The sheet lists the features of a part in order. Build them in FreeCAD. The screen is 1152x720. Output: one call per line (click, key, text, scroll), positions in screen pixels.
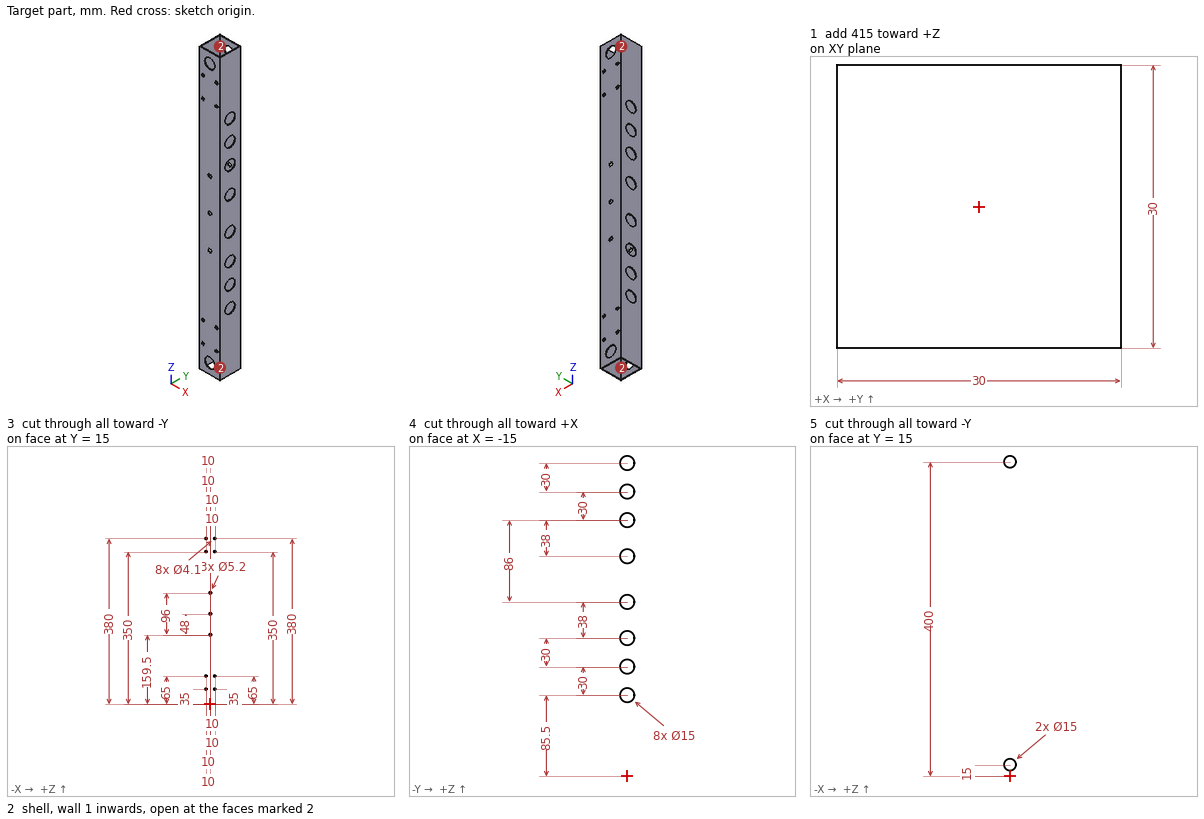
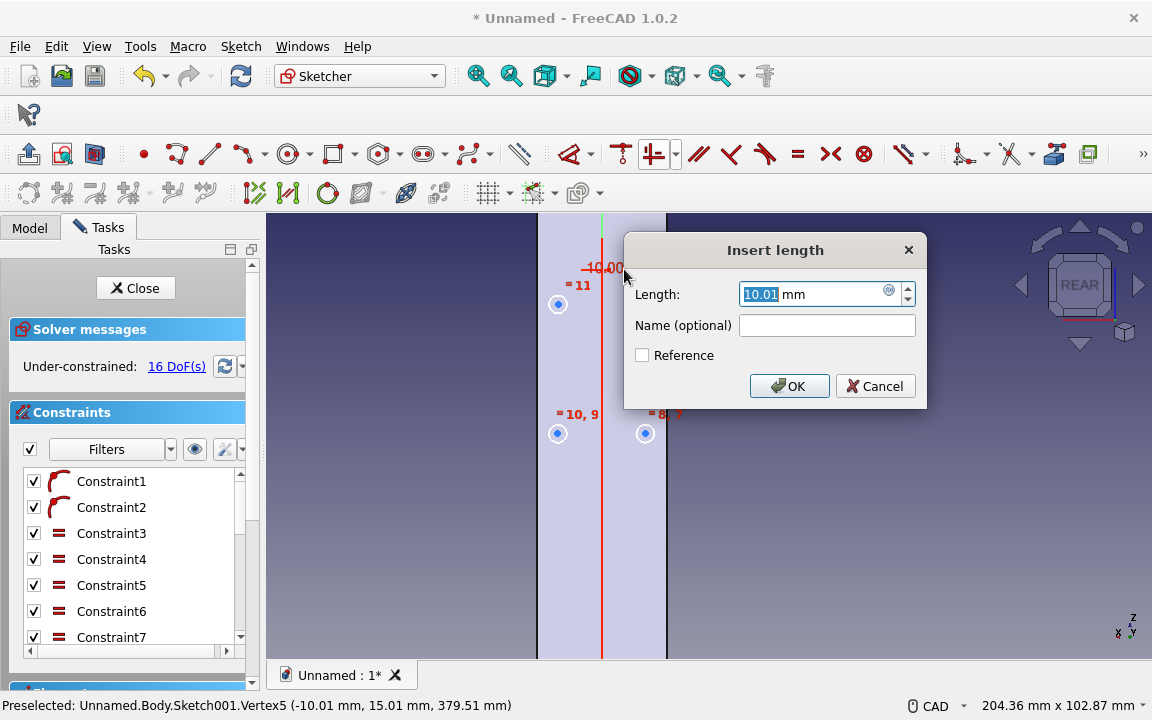
text(10)
key(Return)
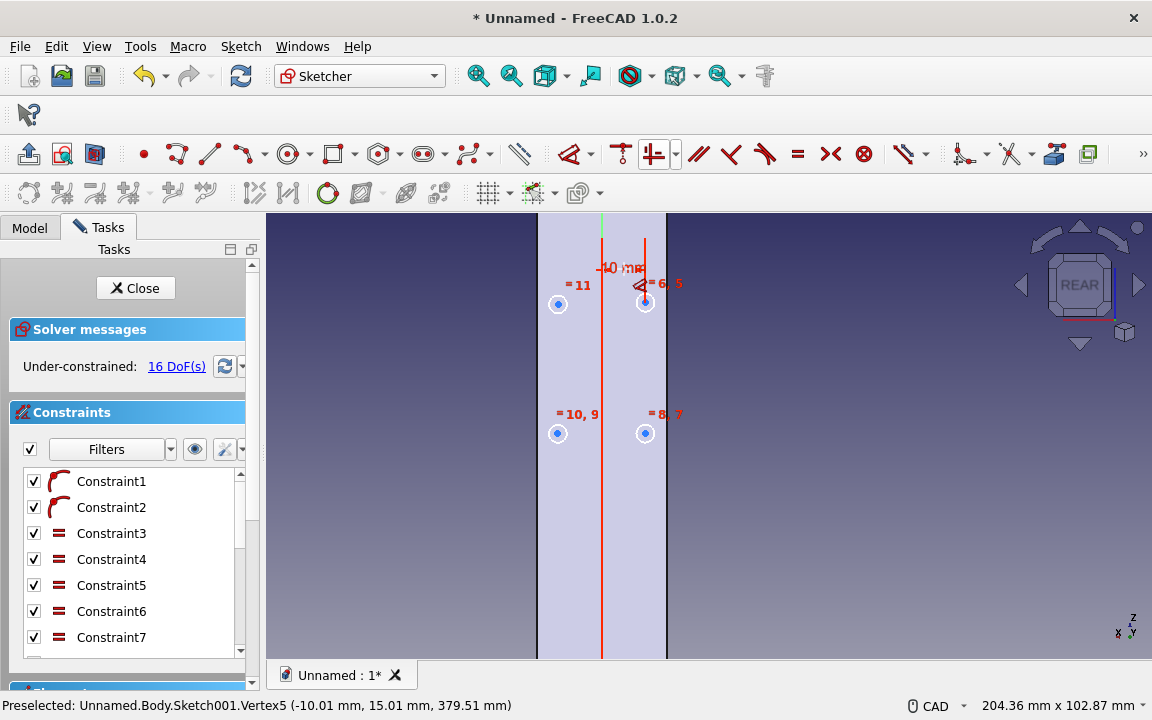
scroll(648, 301, down, 9)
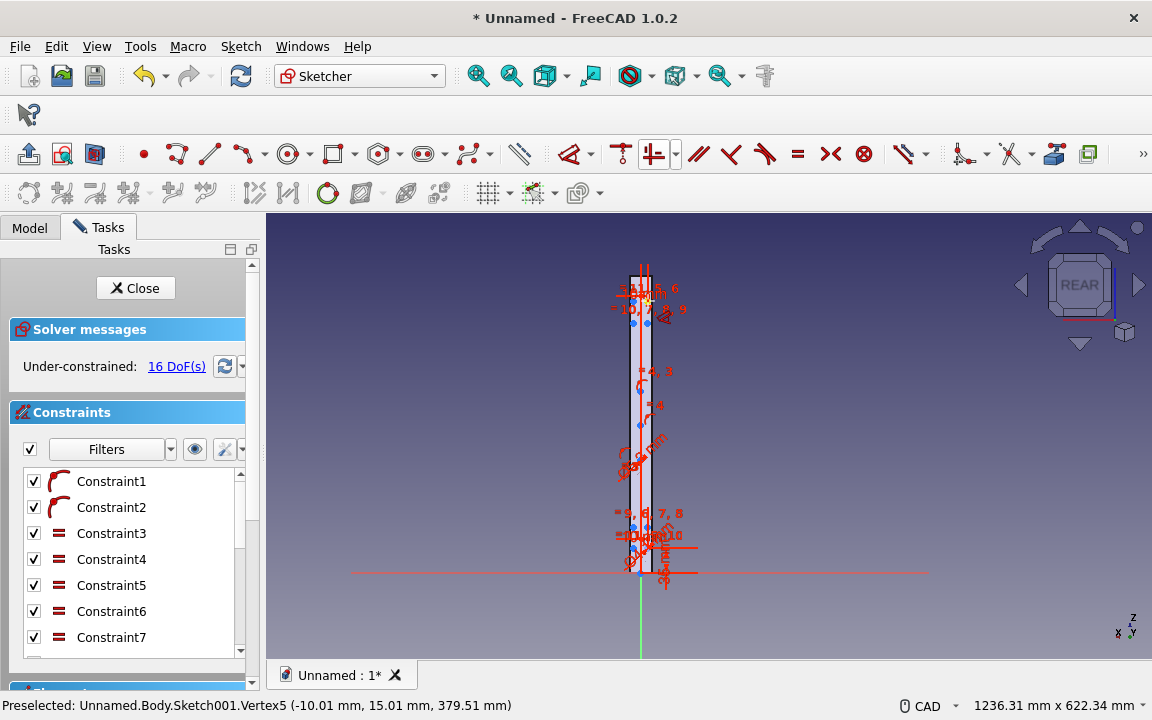
scroll(648, 527, up, 9)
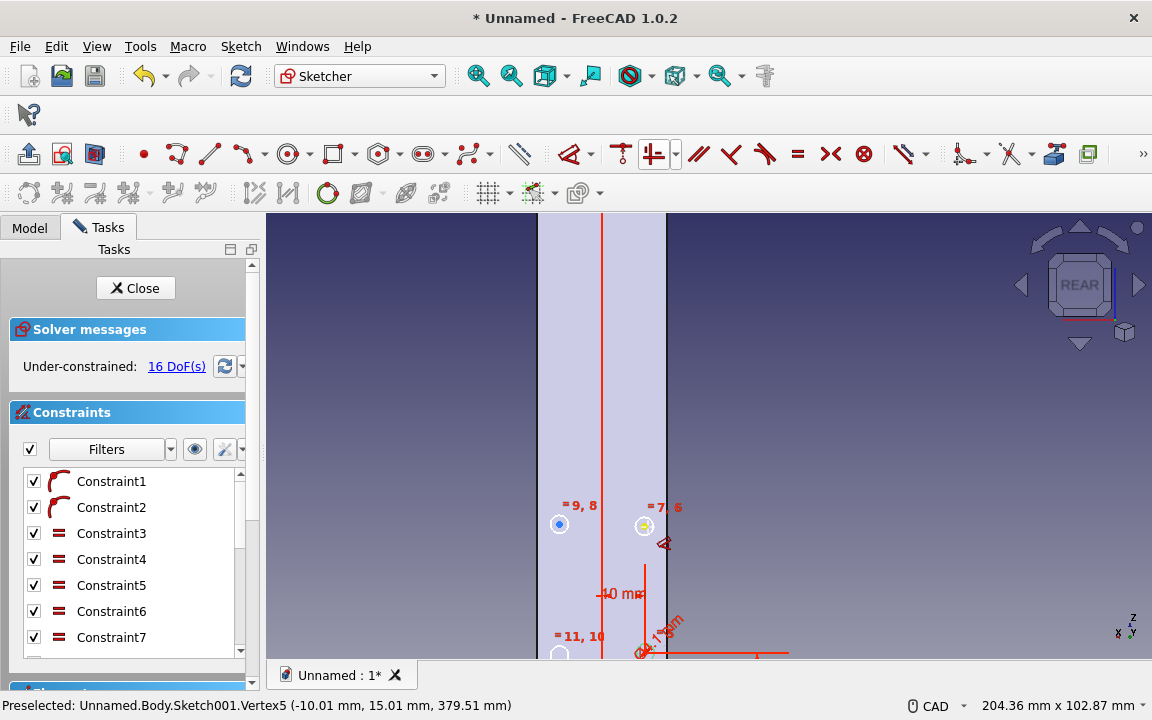
click(644, 526)
click(623, 492)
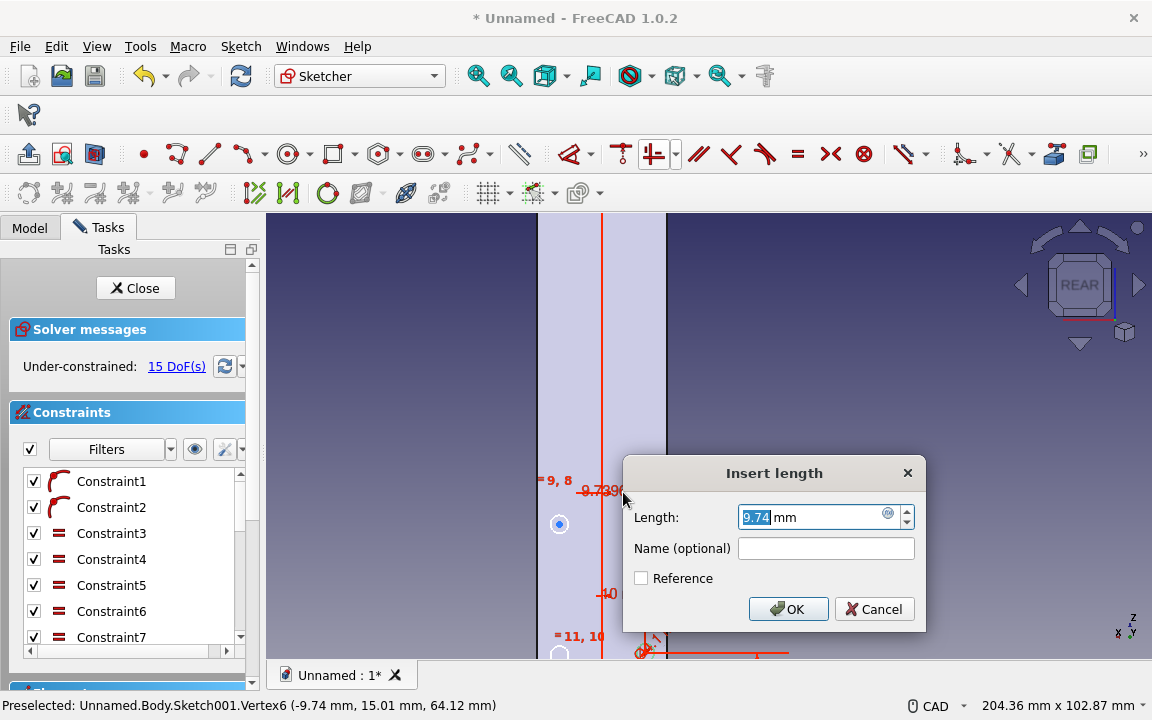
text(10)
key(Return)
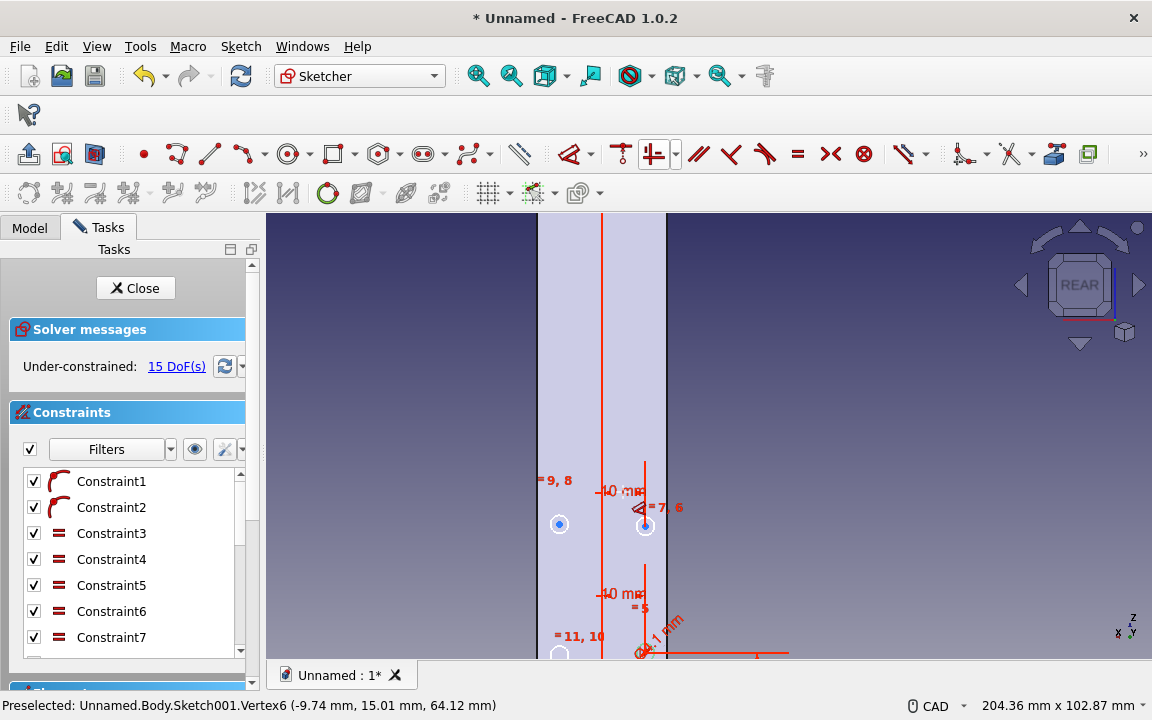
scroll(648, 527, down, 9)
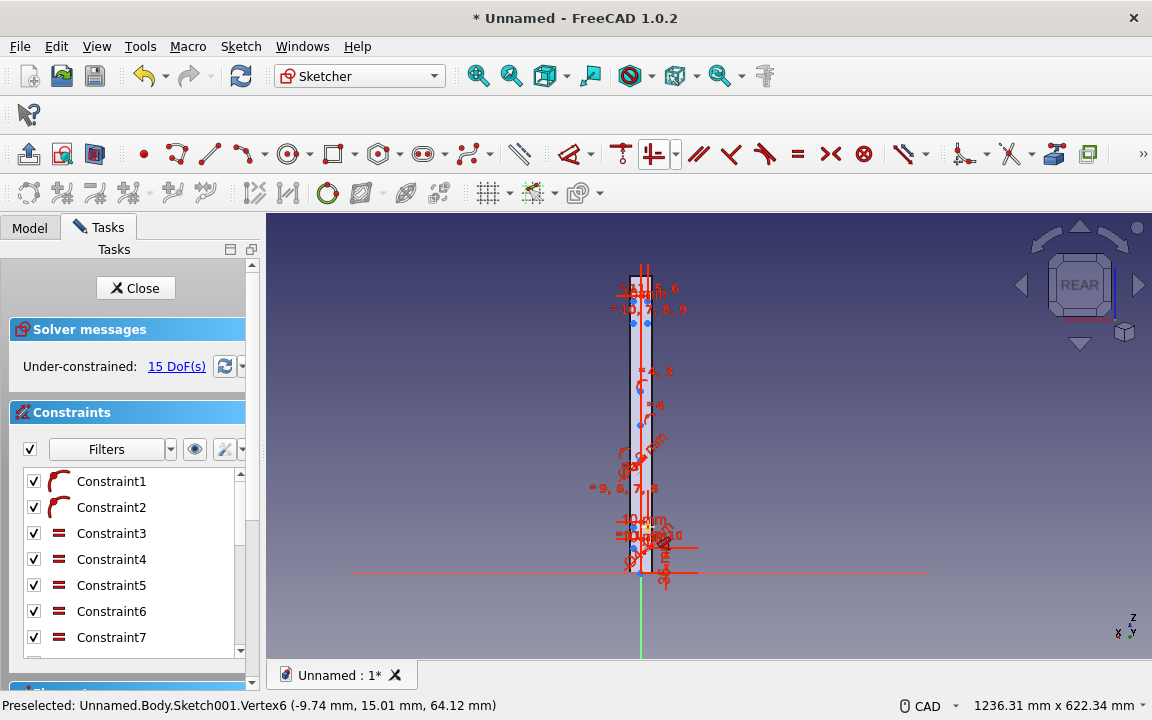
click(648, 527)
click(730, 540)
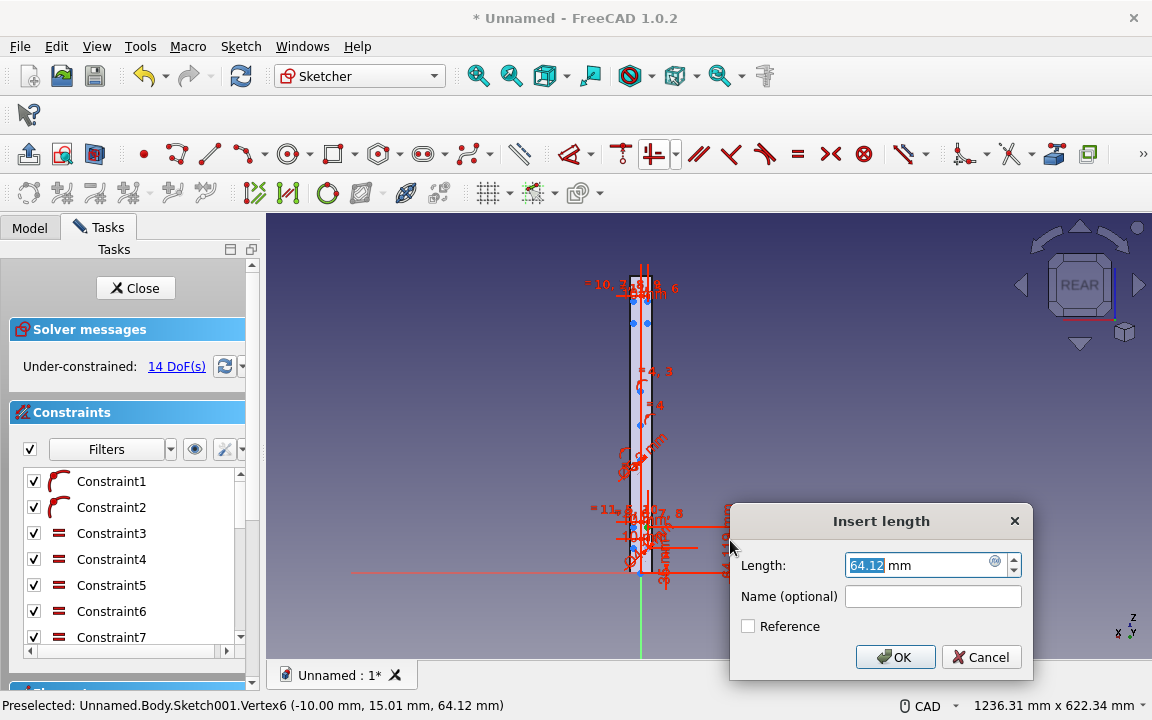
text(65)
key(Return)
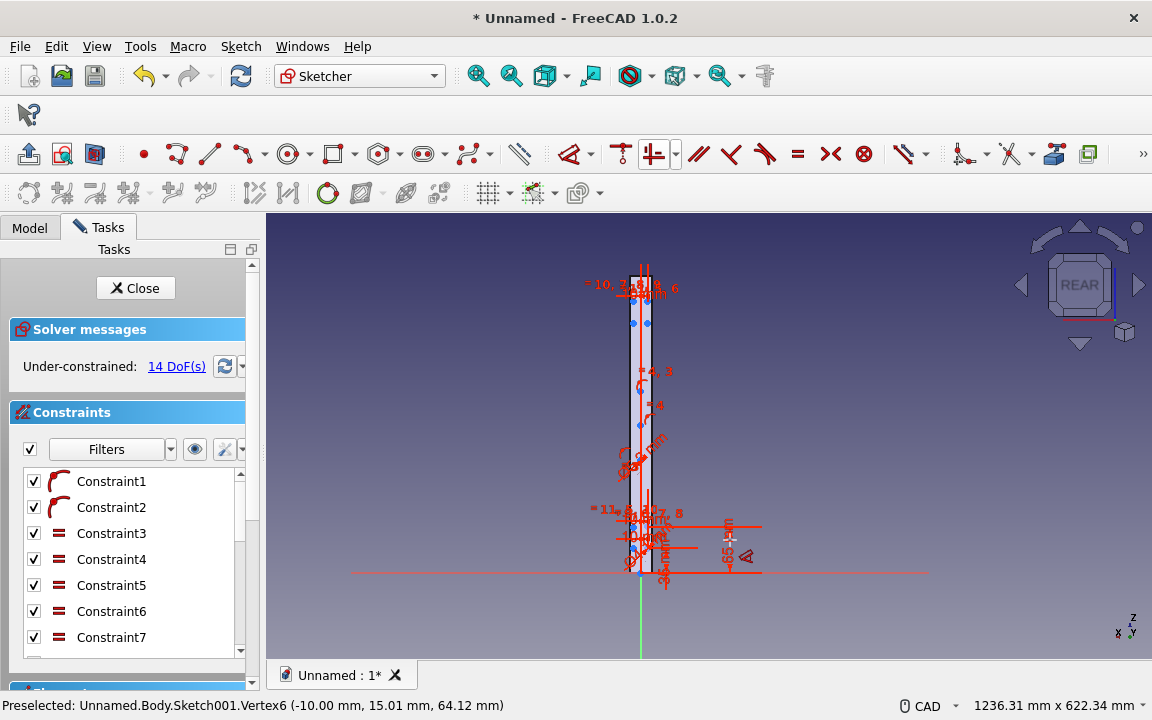
scroll(648, 323, up, 9)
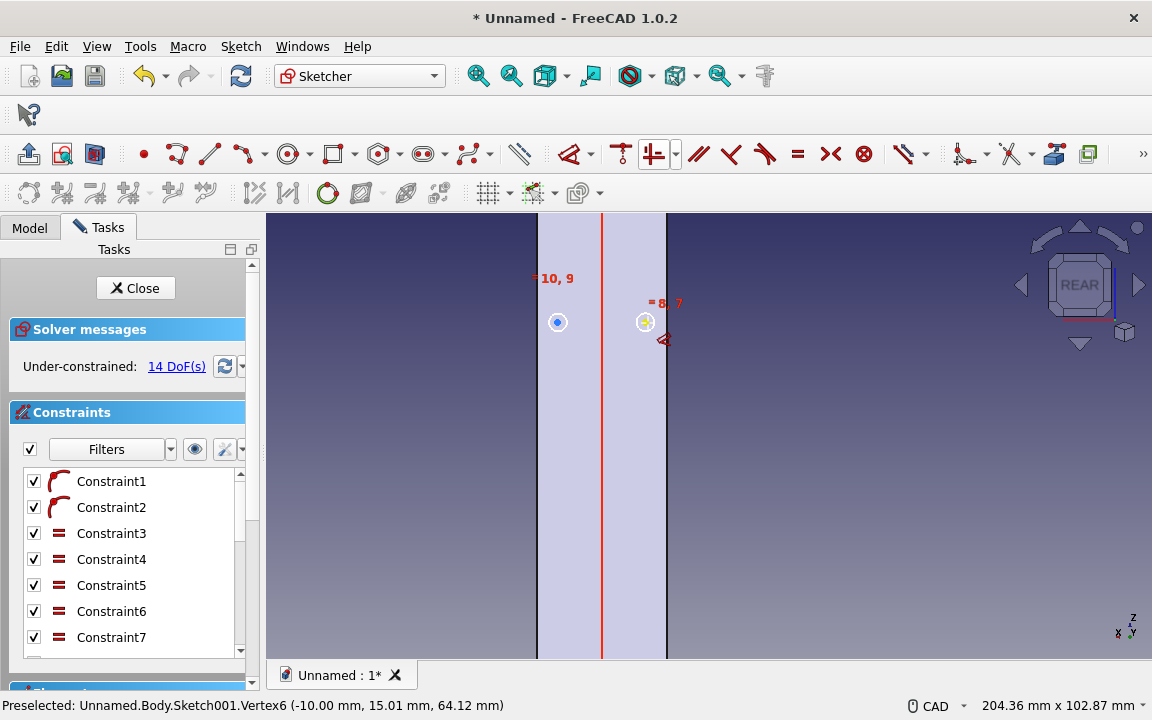
click(645, 322)
click(624, 288)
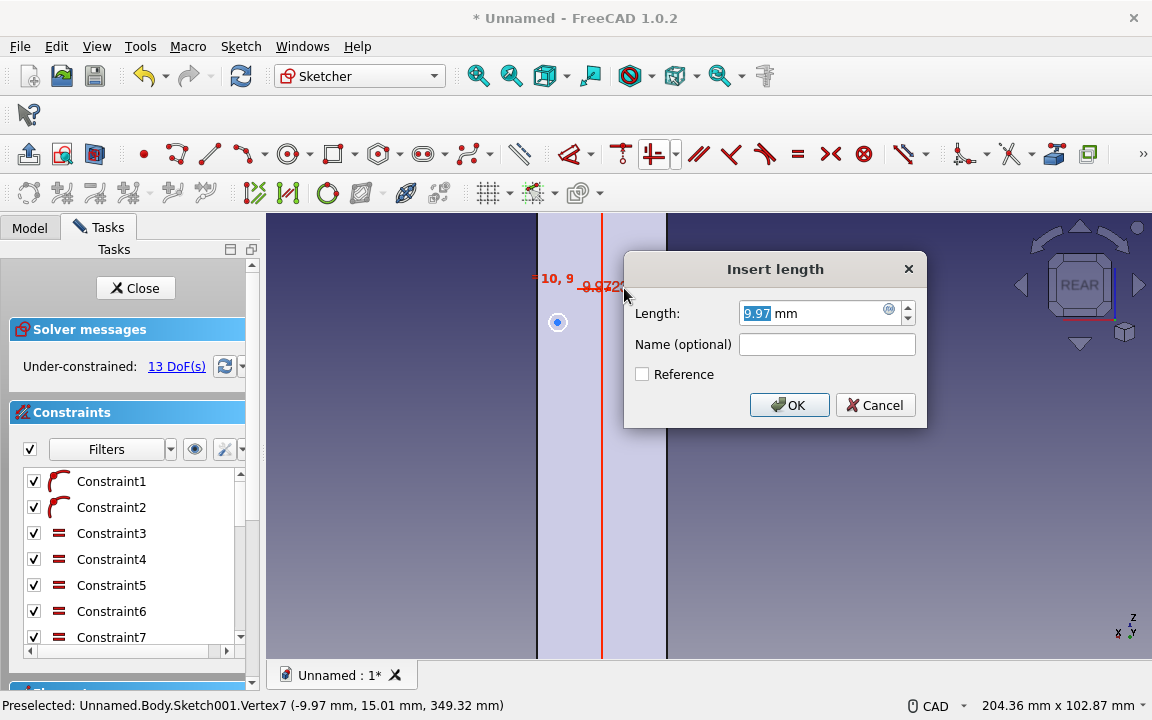
text(10)
key(Return)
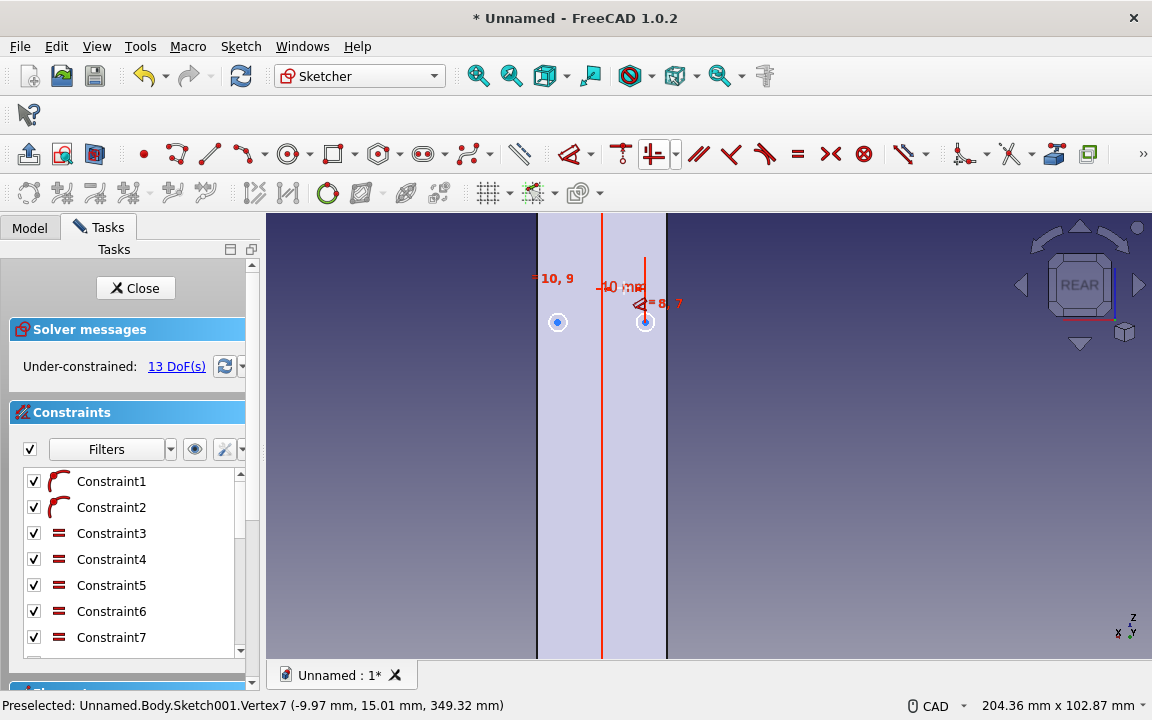
scroll(648, 323, down, 9)